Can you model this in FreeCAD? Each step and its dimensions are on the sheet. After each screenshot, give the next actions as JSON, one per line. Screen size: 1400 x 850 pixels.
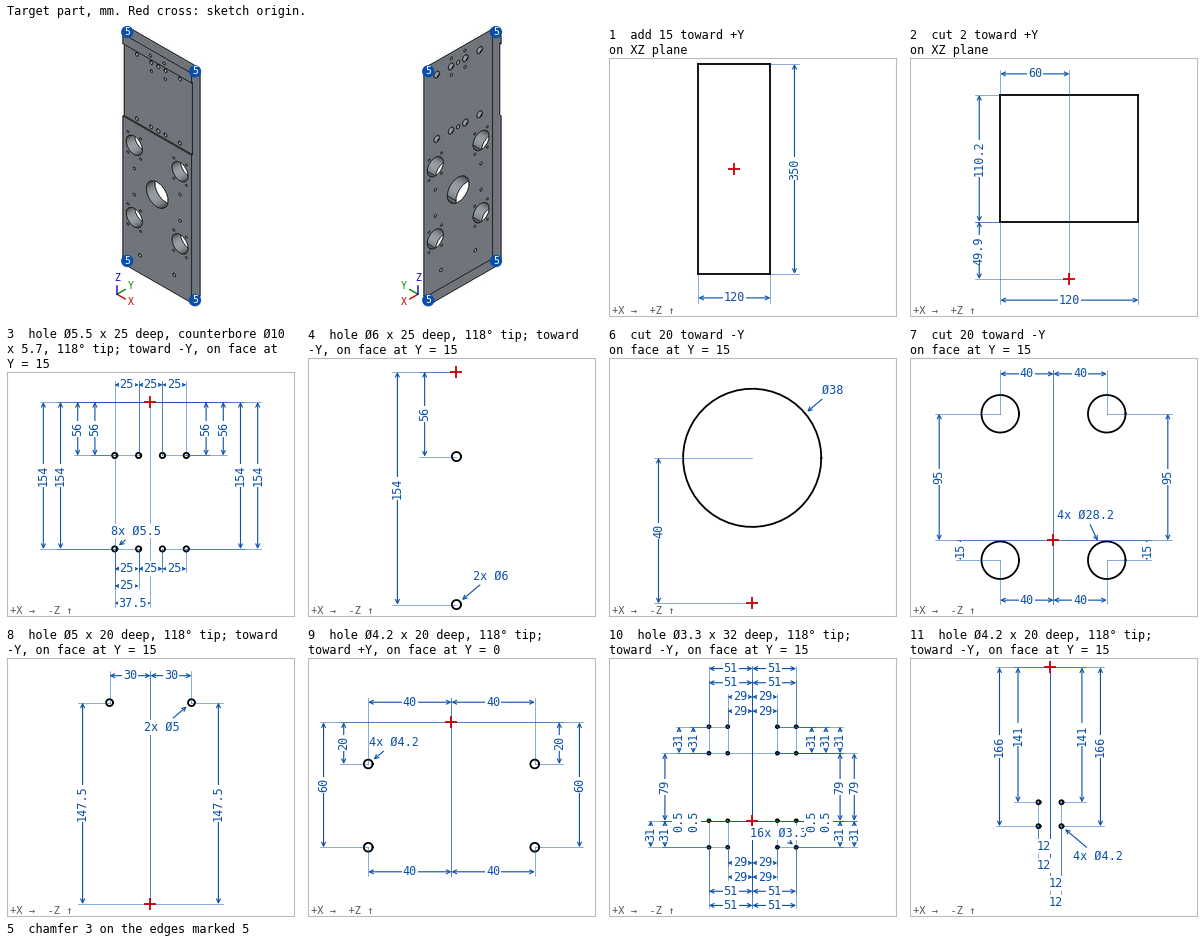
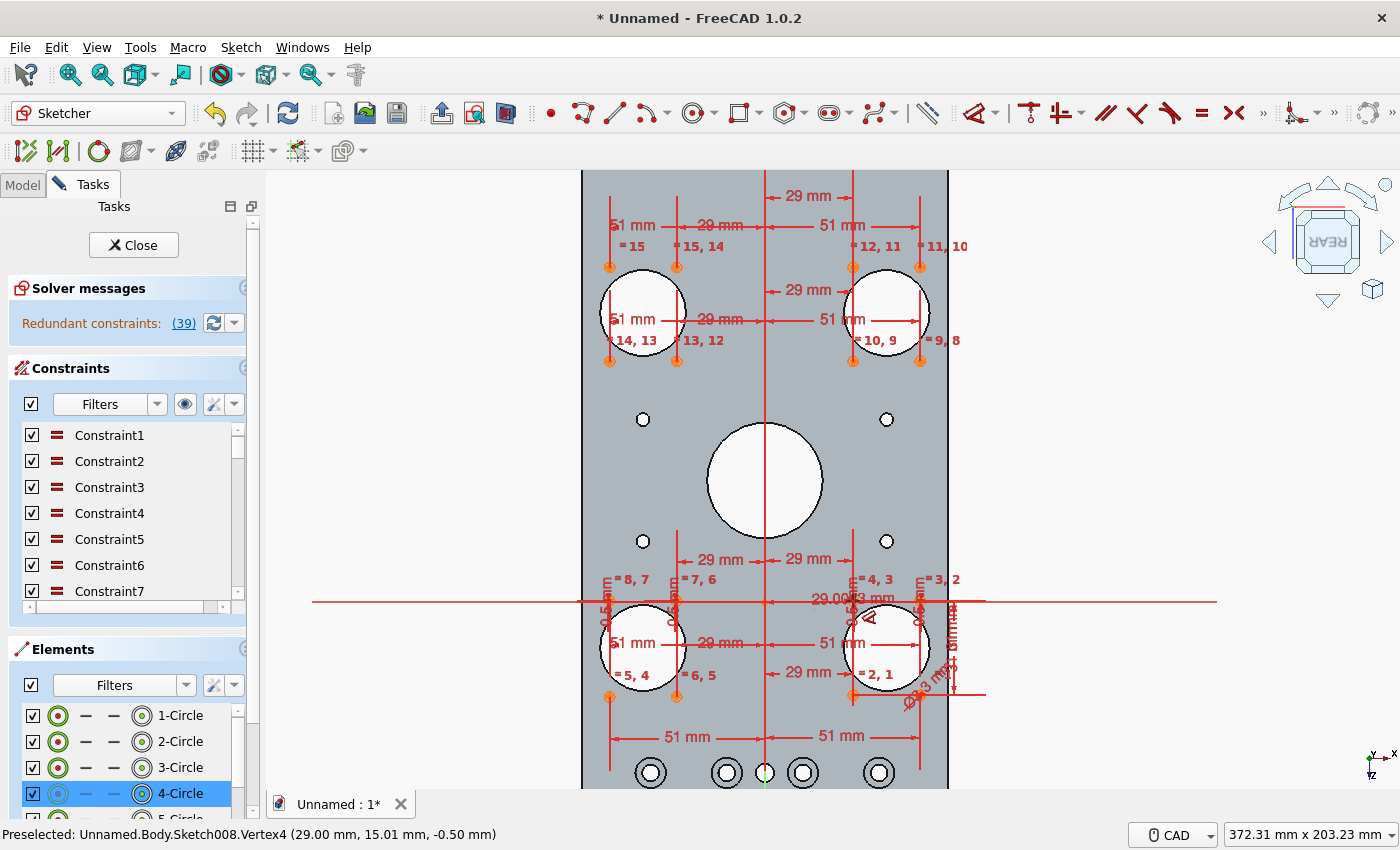
{"action": "left_click", "coordinate": [610, 697]}
{"action": "left_click", "coordinate": [576, 671]}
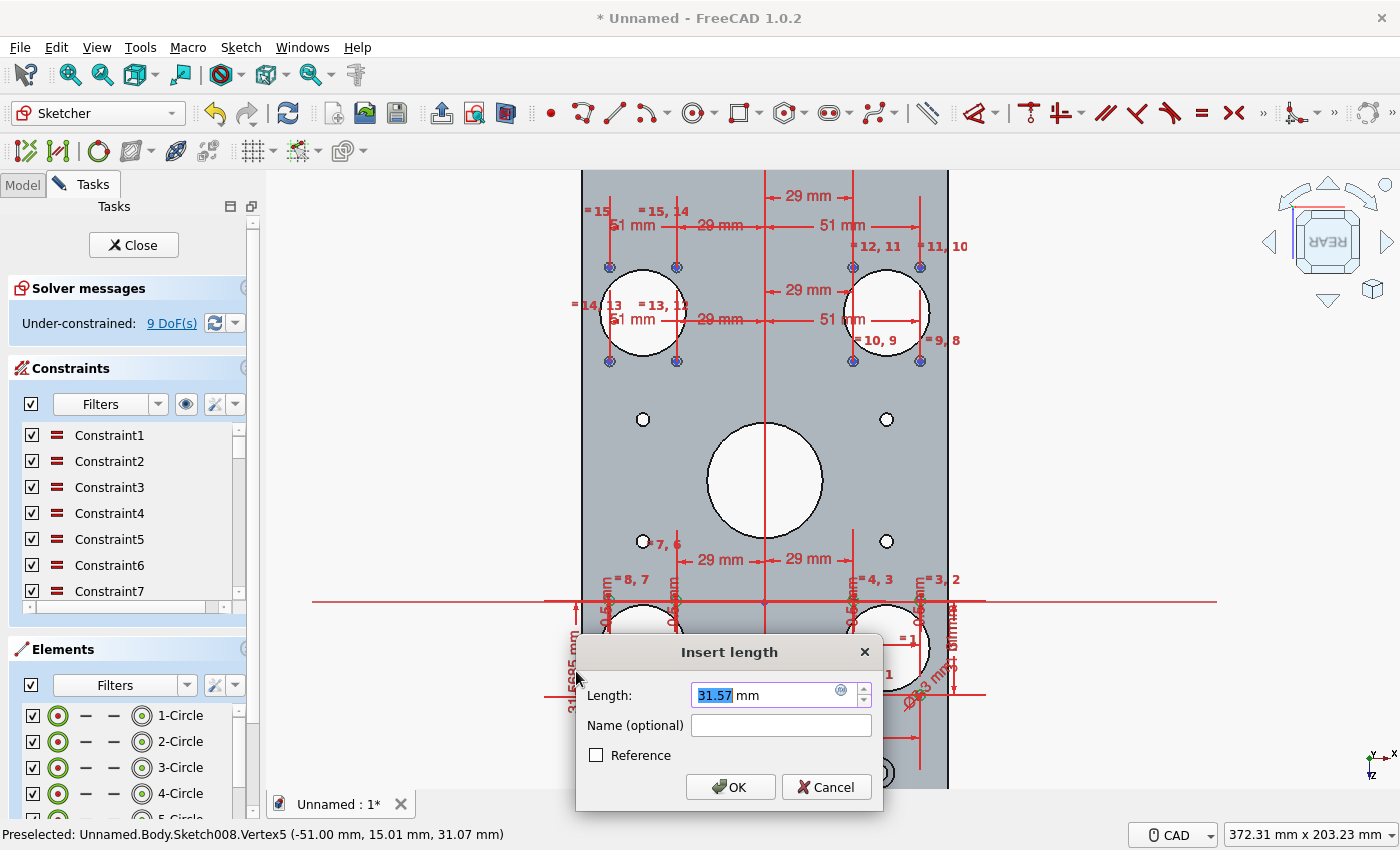
{"action": "type", "text": "31"}
{"action": "key", "text": "Return"}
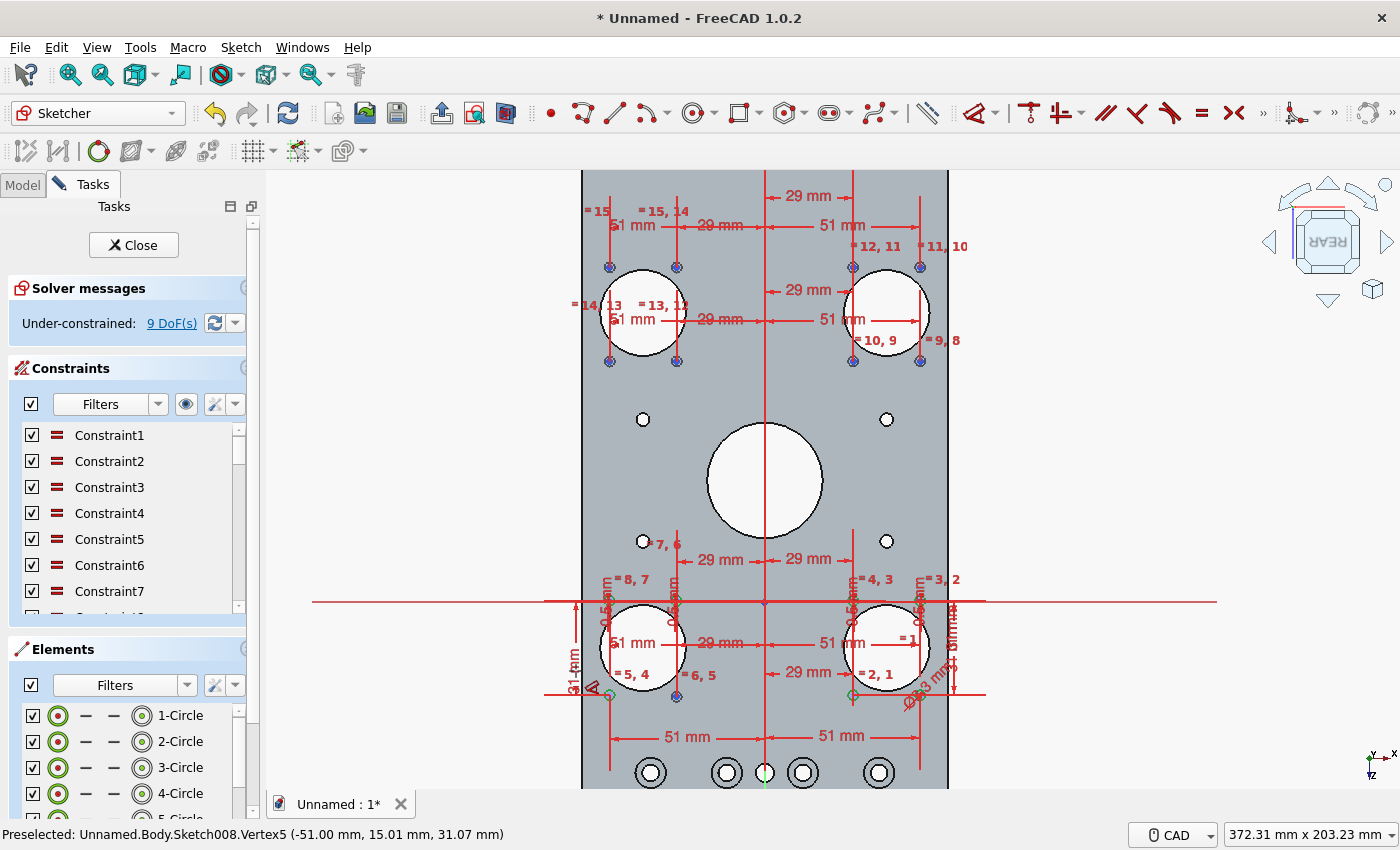
{"action": "left_click", "coordinate": [853, 601]}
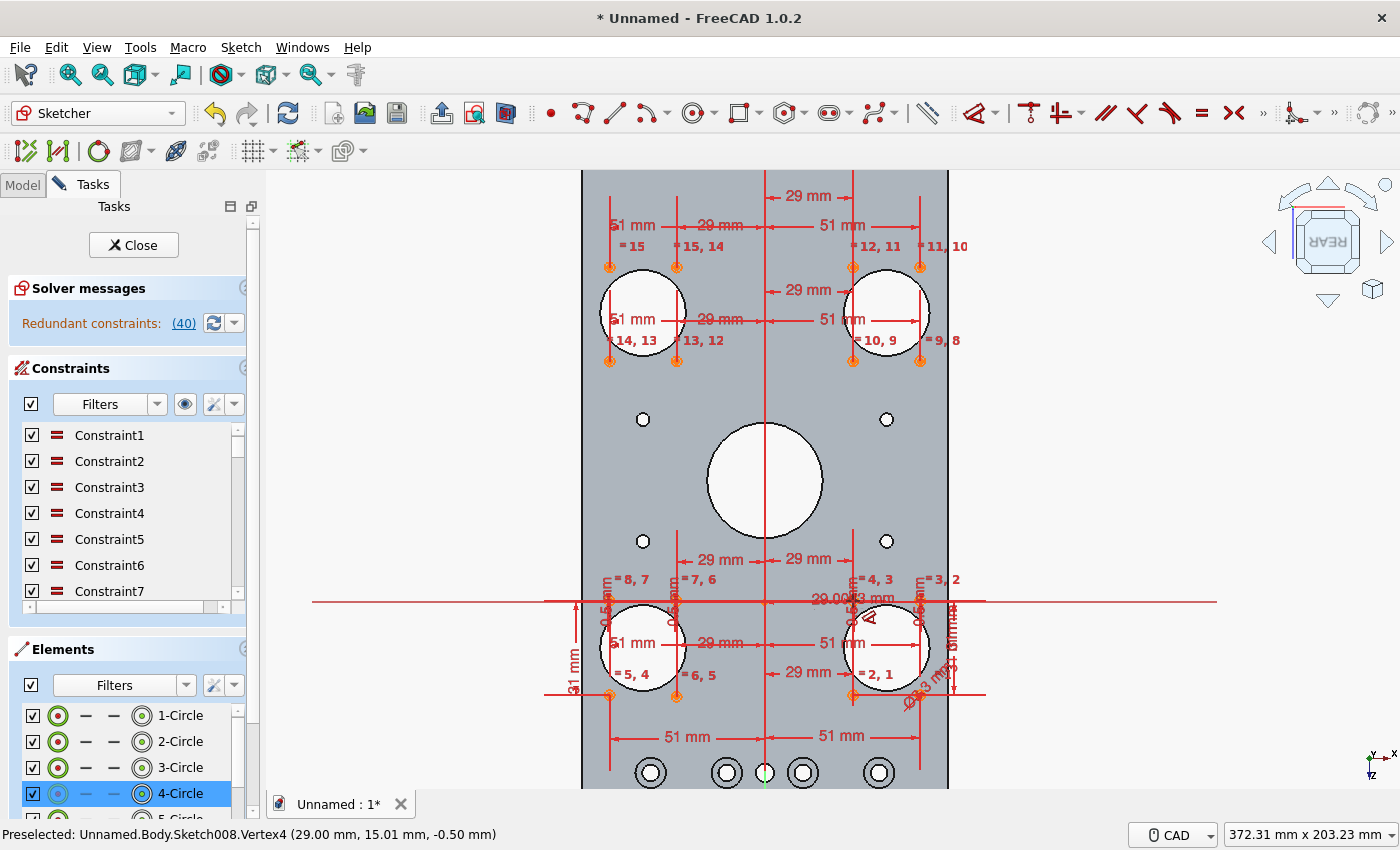
{"action": "left_click", "coordinate": [677, 697]}
{"action": "left_click", "coordinate": [547, 649]}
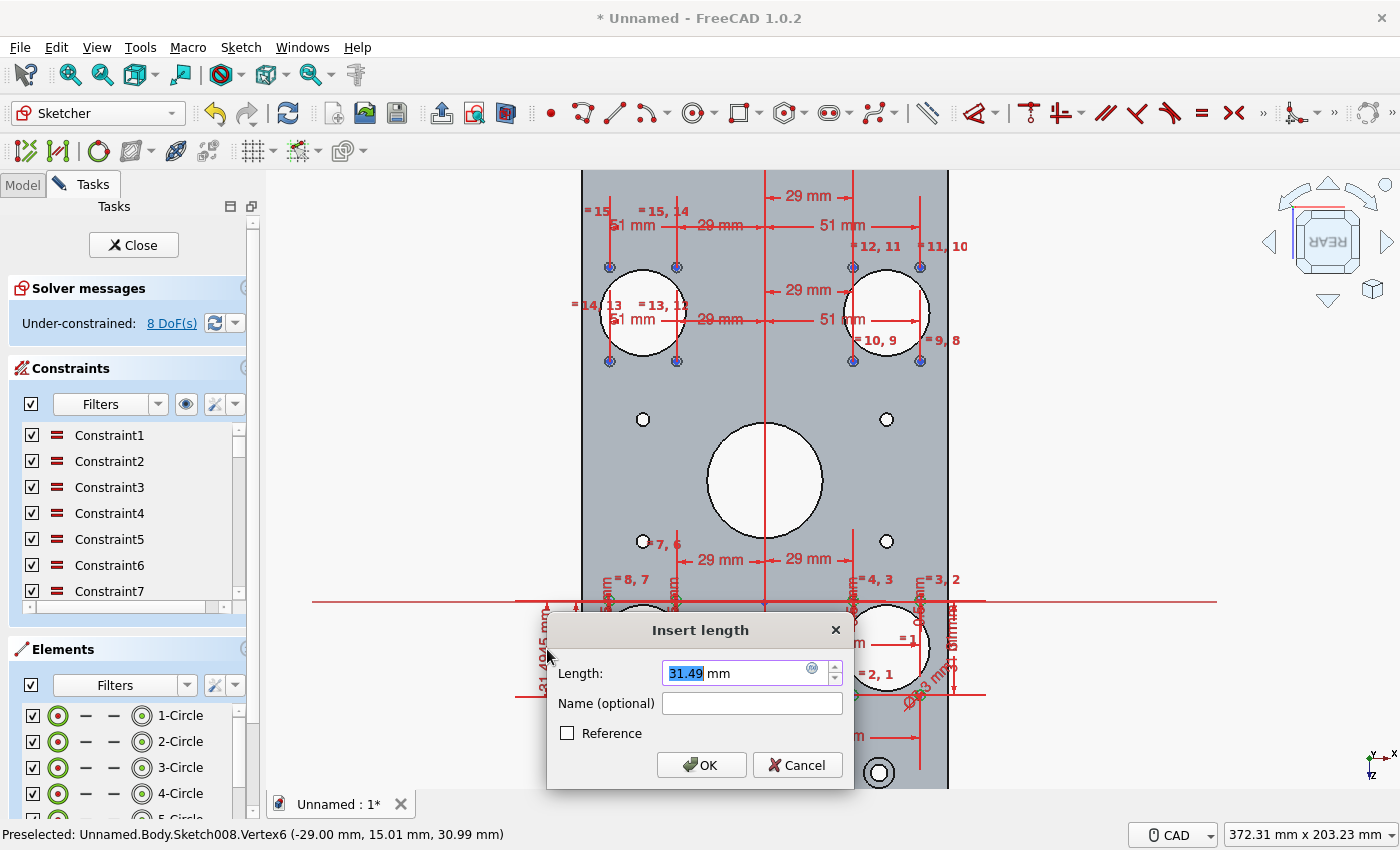
{"action": "type", "text": "31"}
{"action": "key", "text": "Return"}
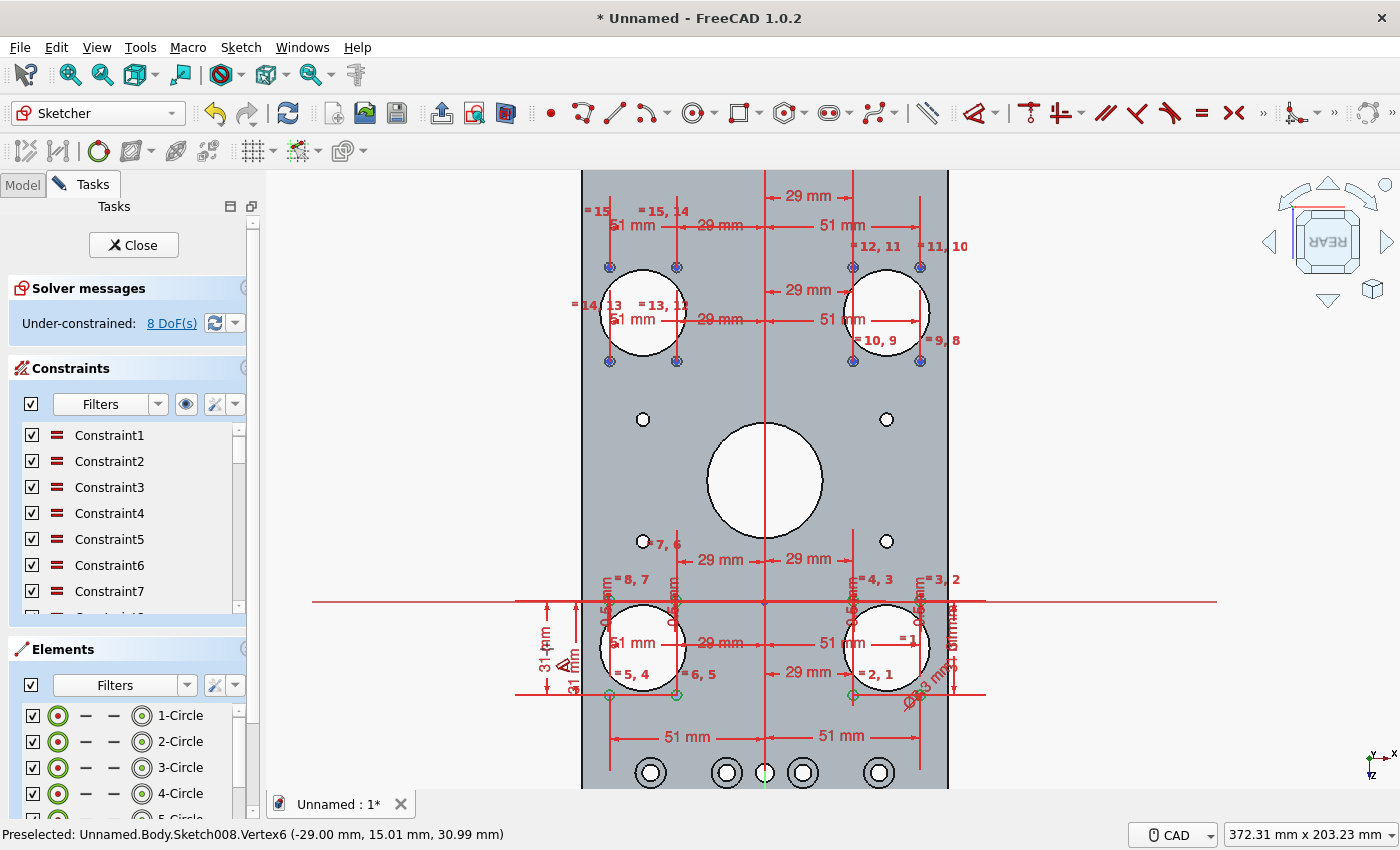
{"action": "left_click", "coordinate": [920, 601]}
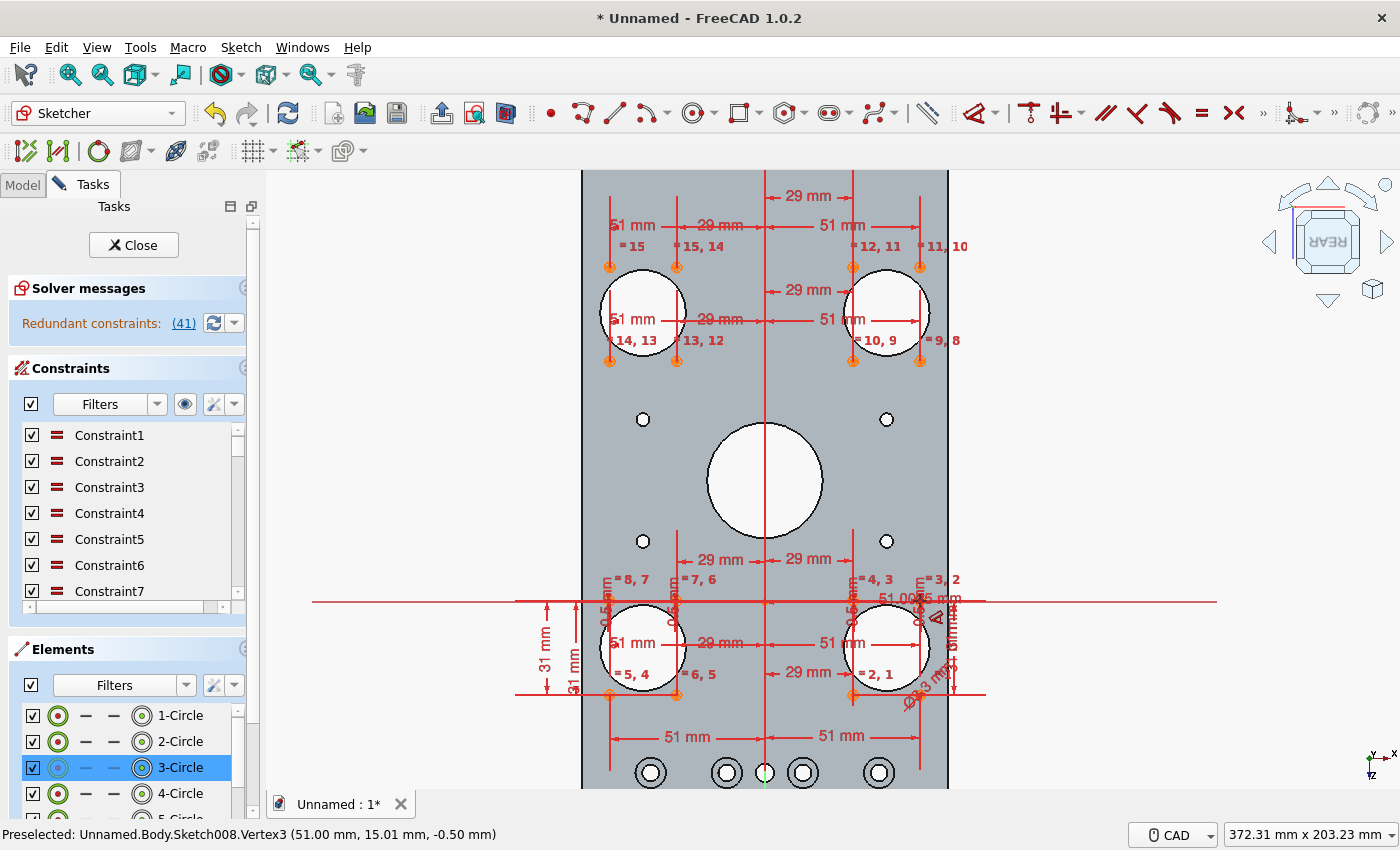
{"action": "left_click", "coordinate": [920, 361]}
{"action": "left_click", "coordinate": [954, 481]}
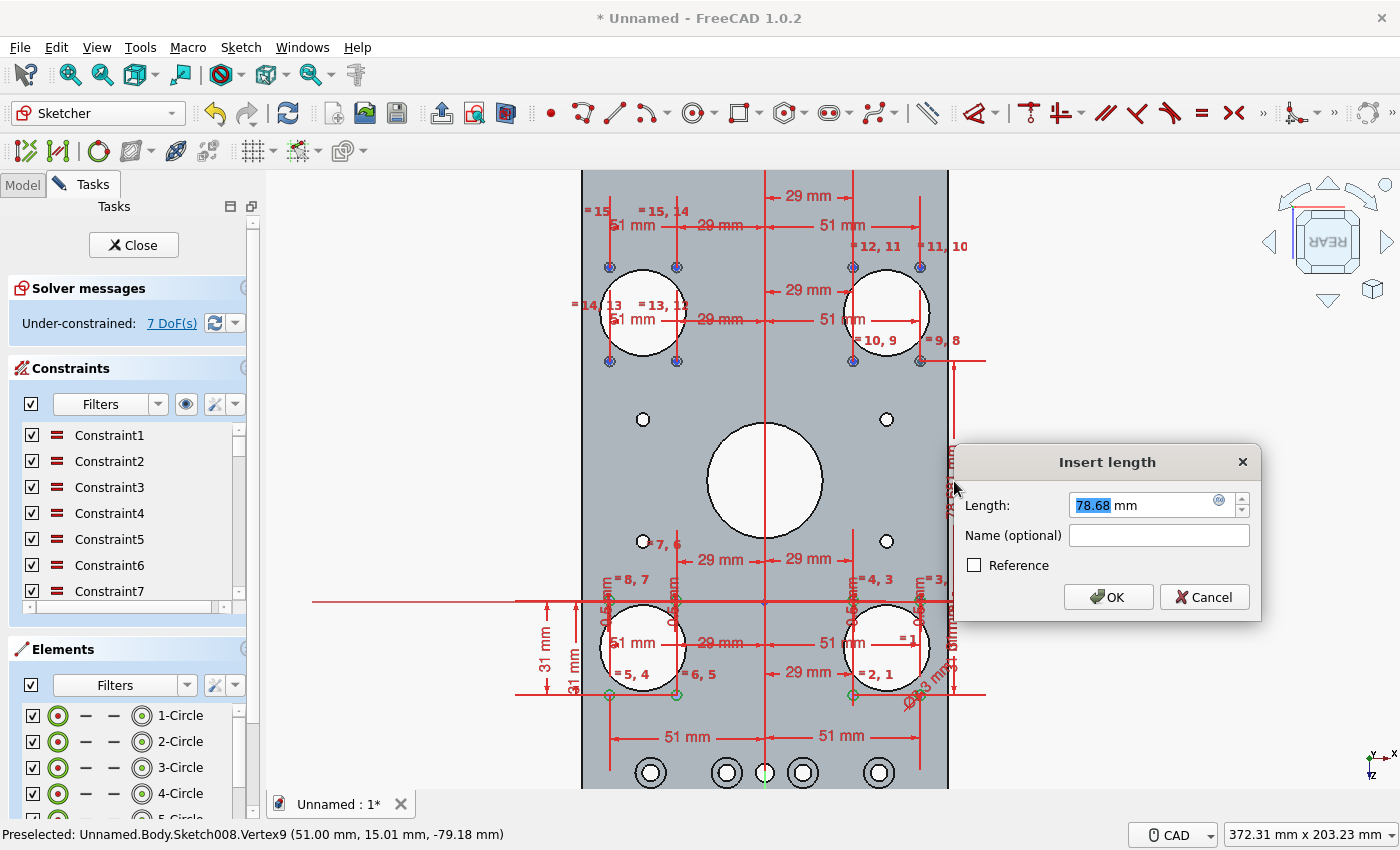
{"action": "type", "text": "79"}
{"action": "key", "text": "Return"}